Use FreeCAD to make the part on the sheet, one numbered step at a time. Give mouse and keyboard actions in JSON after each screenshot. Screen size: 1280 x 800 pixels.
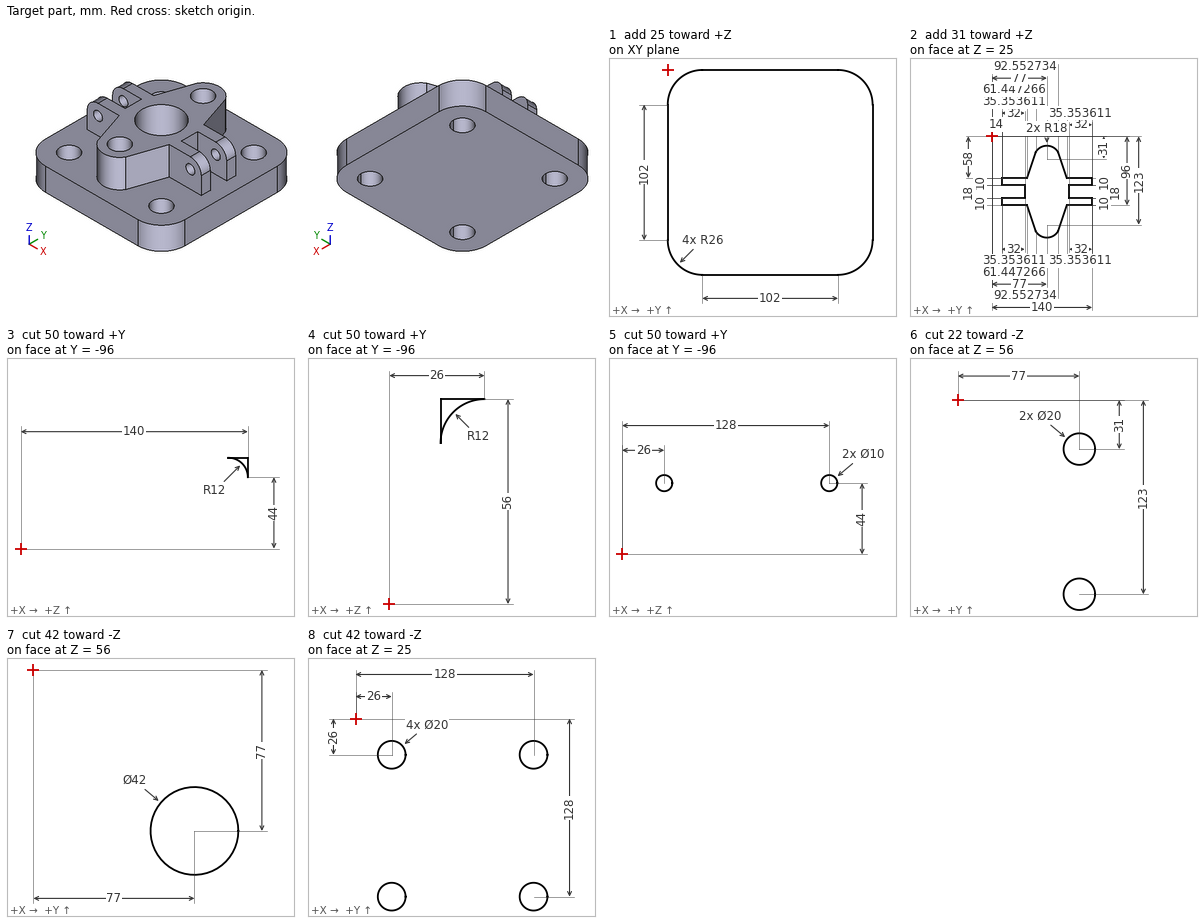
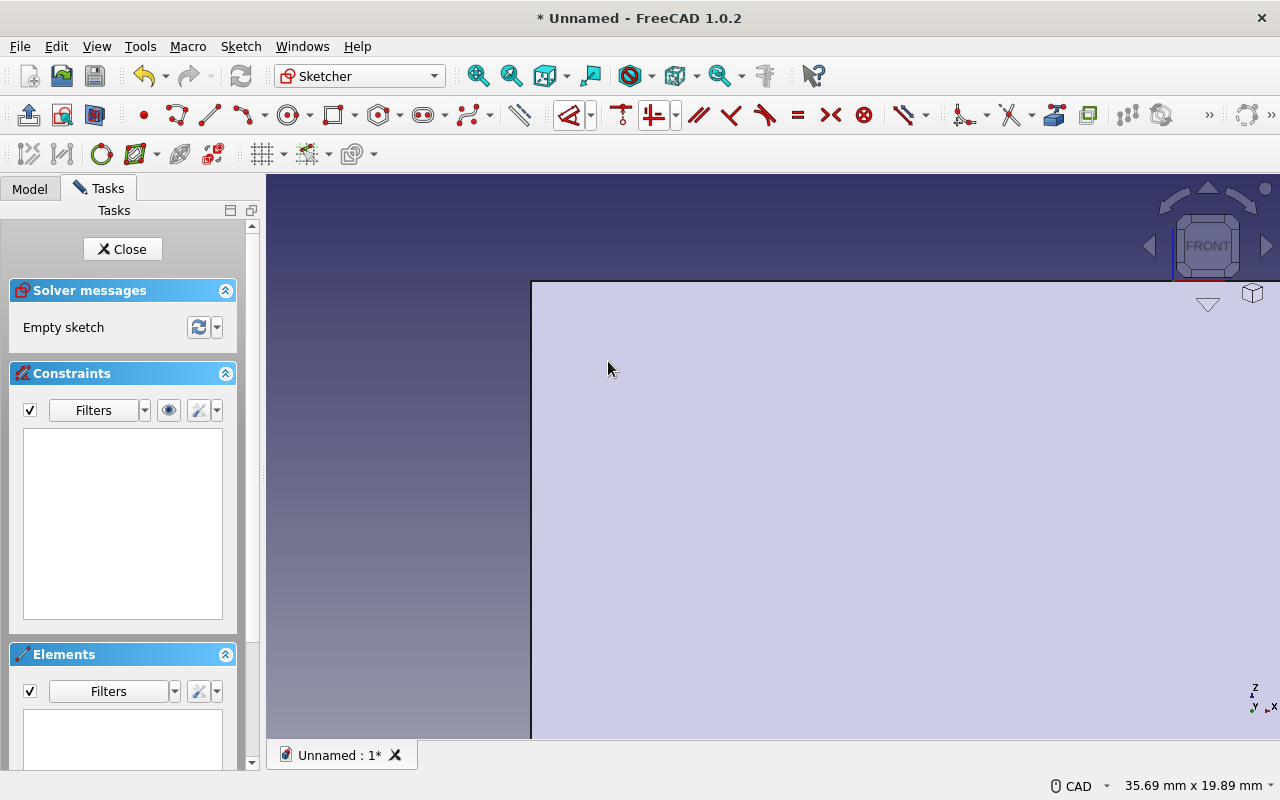
{"action": "left_click", "coordinate": [177, 116]}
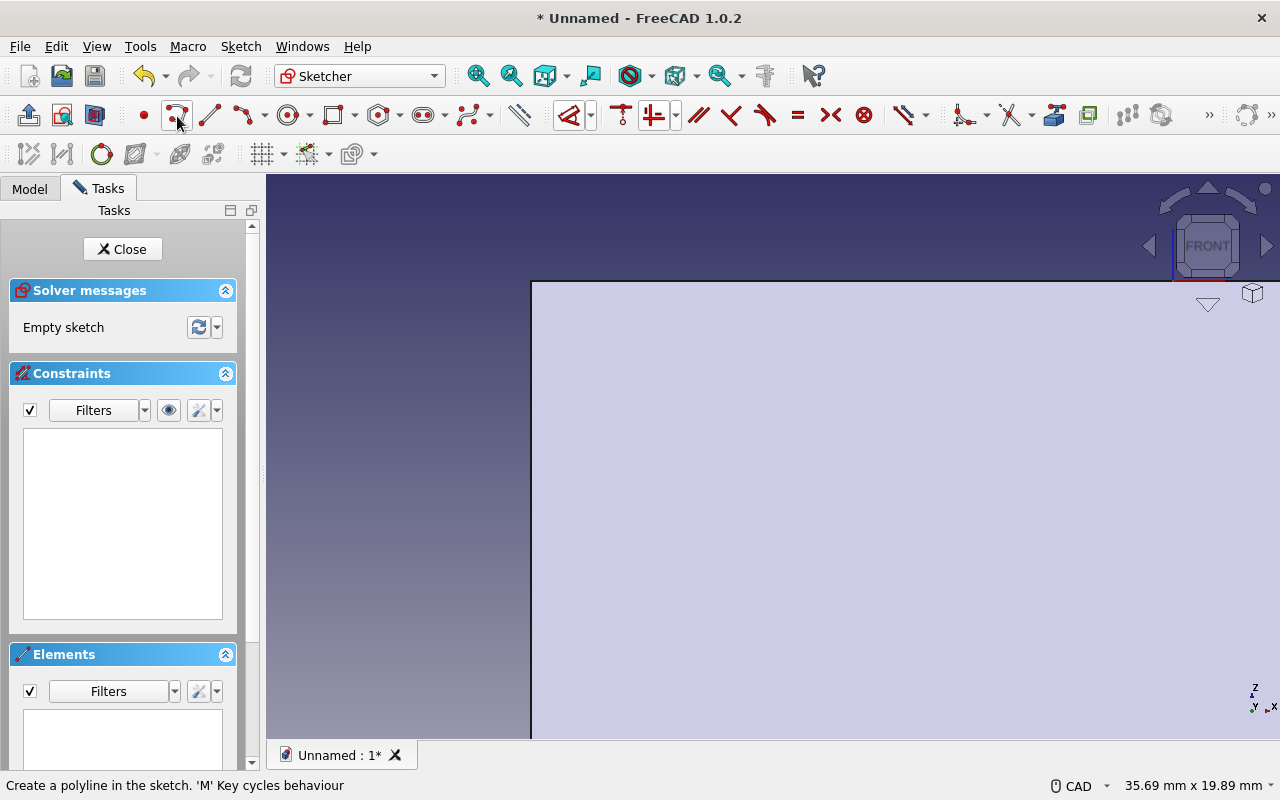
{"action": "left_click", "coordinate": [872, 281]}
{"action": "left_click", "coordinate": [531, 281]}
{"action": "left_click", "coordinate": [531, 622]}
{"action": "right_click", "coordinate": [531, 622]}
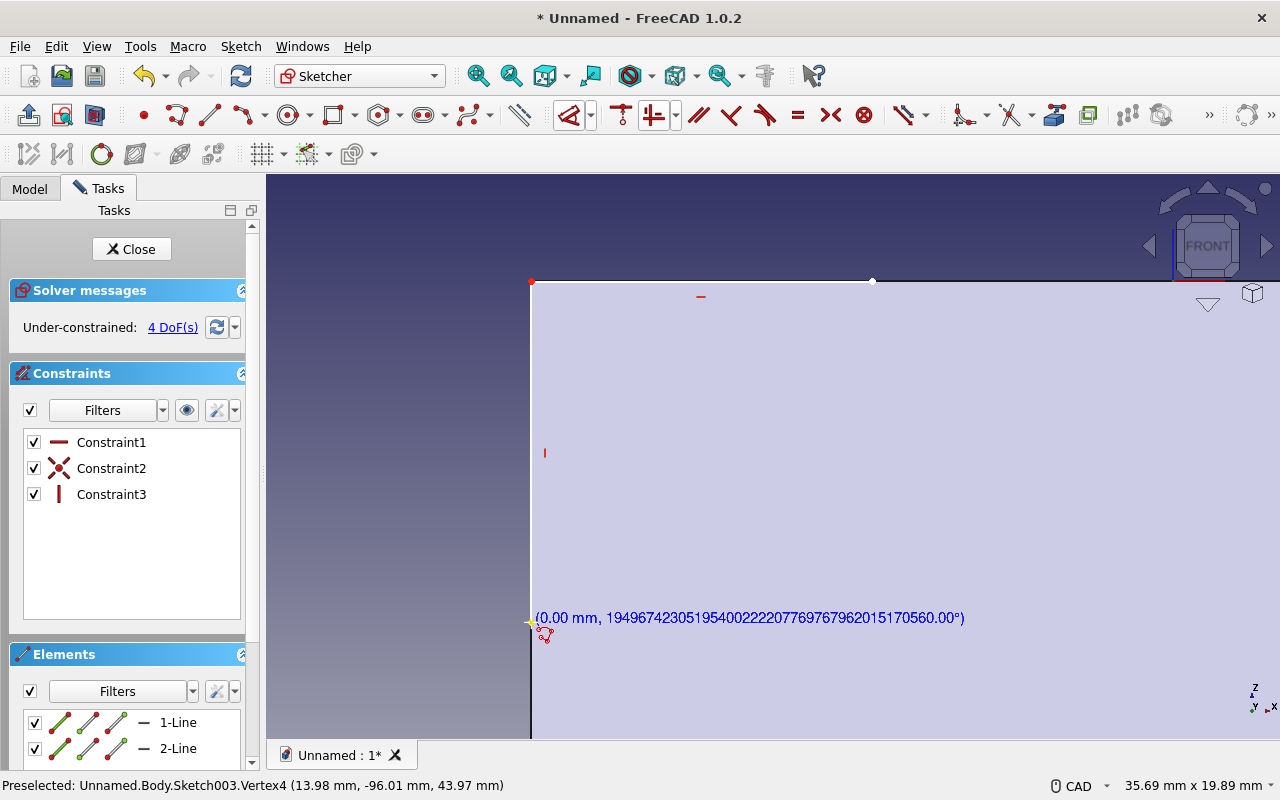
{"action": "left_click", "coordinate": [242, 116]}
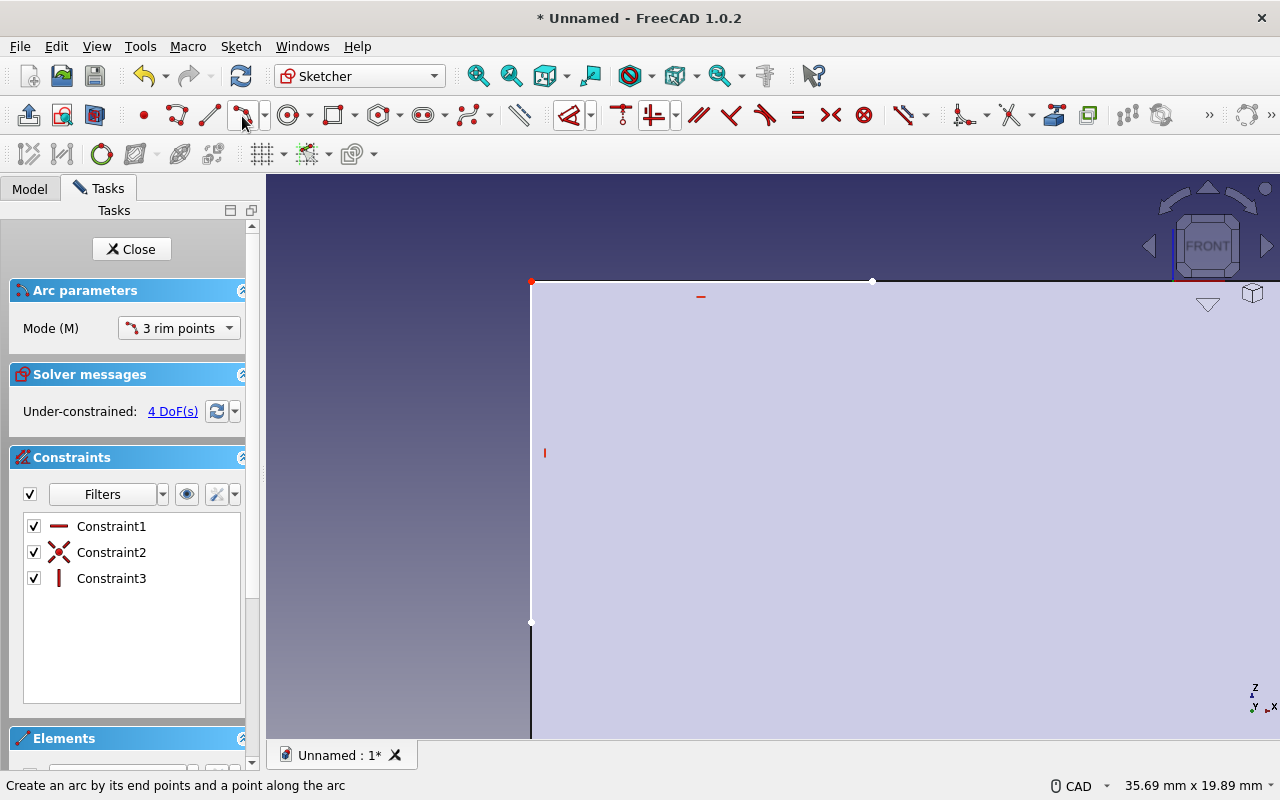
{"action": "left_click", "coordinate": [531, 623]}
{"action": "left_click", "coordinate": [872, 282]}
{"action": "left_click", "coordinate": [631, 381]}
{"action": "key", "text": "Escape"}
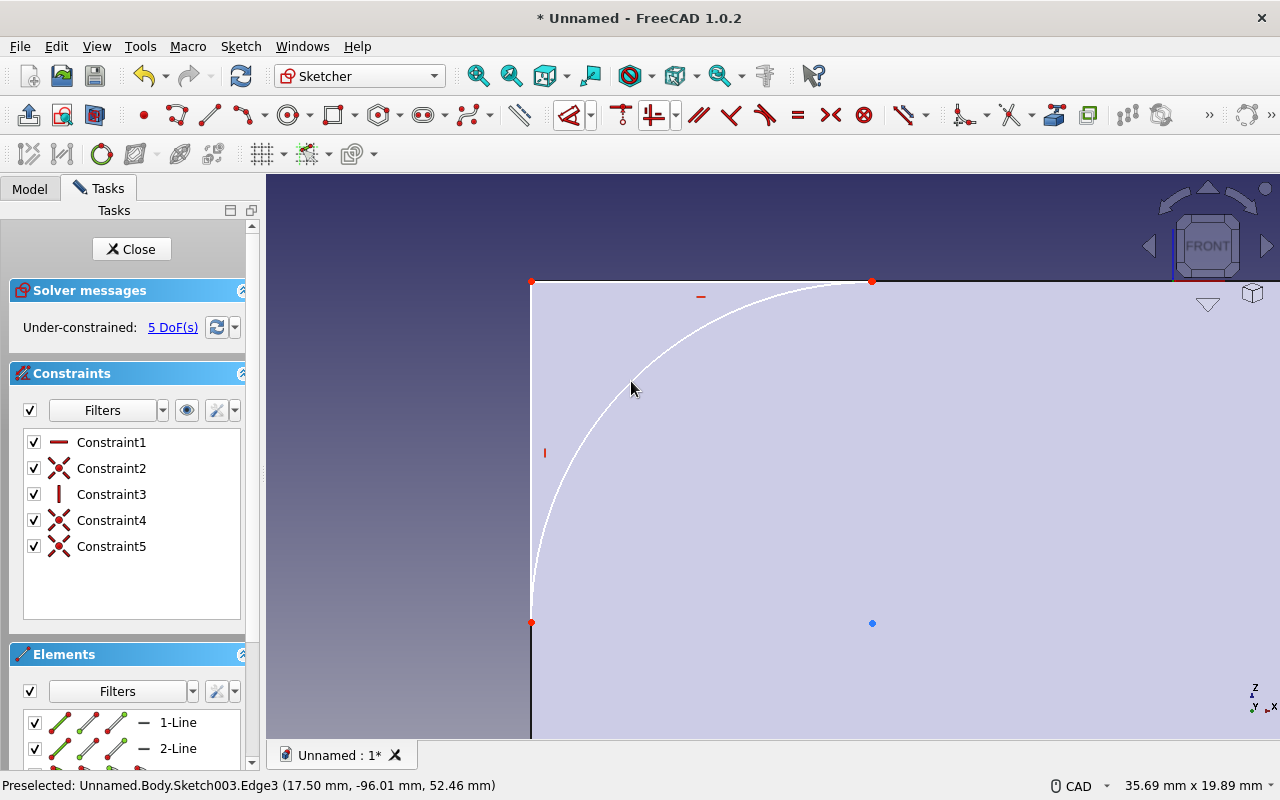
{"action": "left_click", "coordinate": [770, 282]}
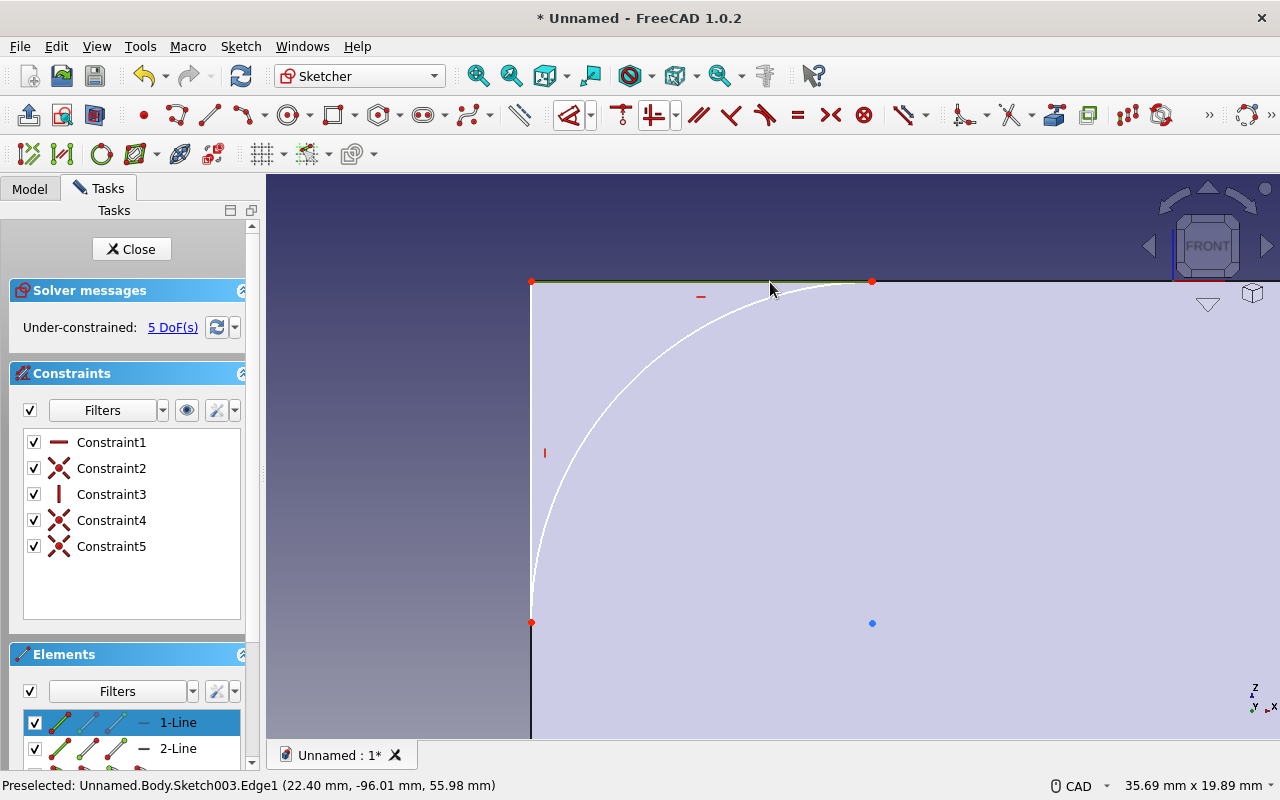
{"action": "left_click", "coordinate": [717, 319]}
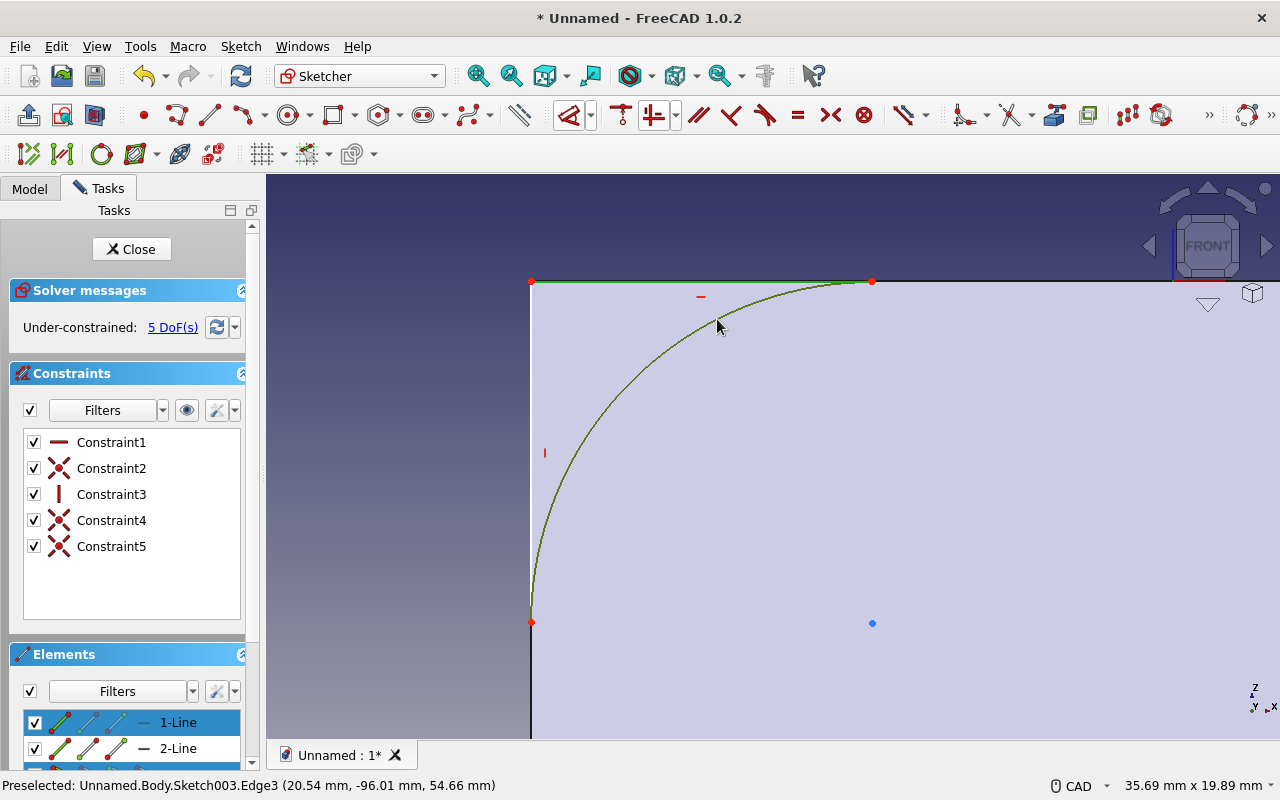
{"action": "left_click", "coordinate": [765, 116]}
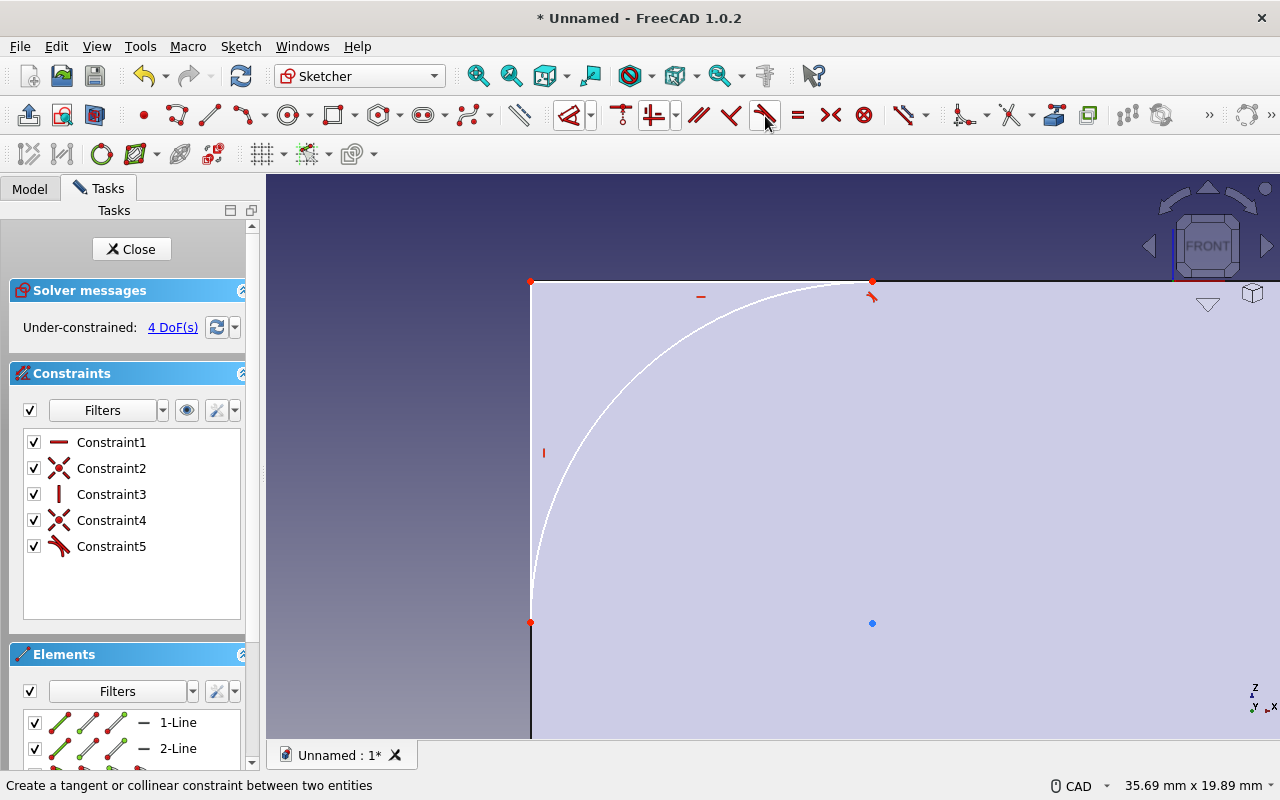
{"action": "left_click", "coordinate": [531, 384]}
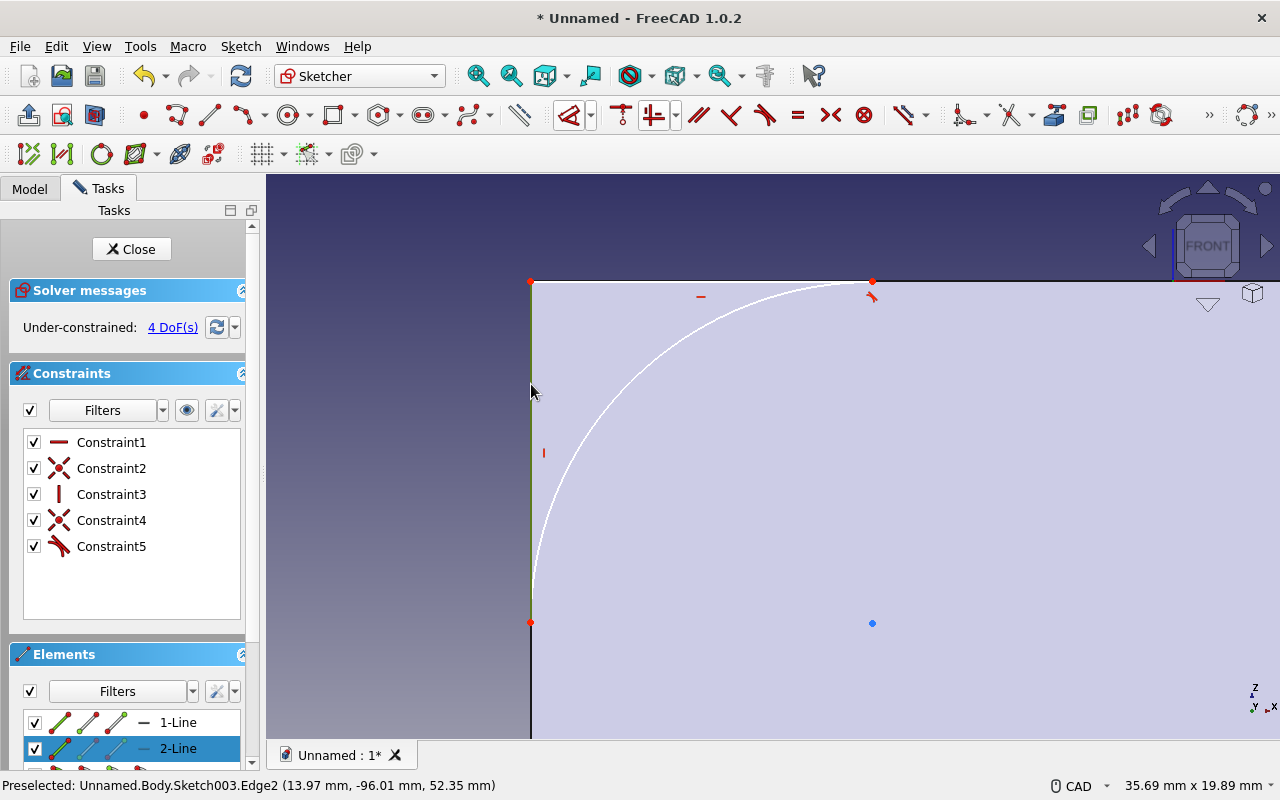
{"action": "left_click", "coordinate": [717, 319]}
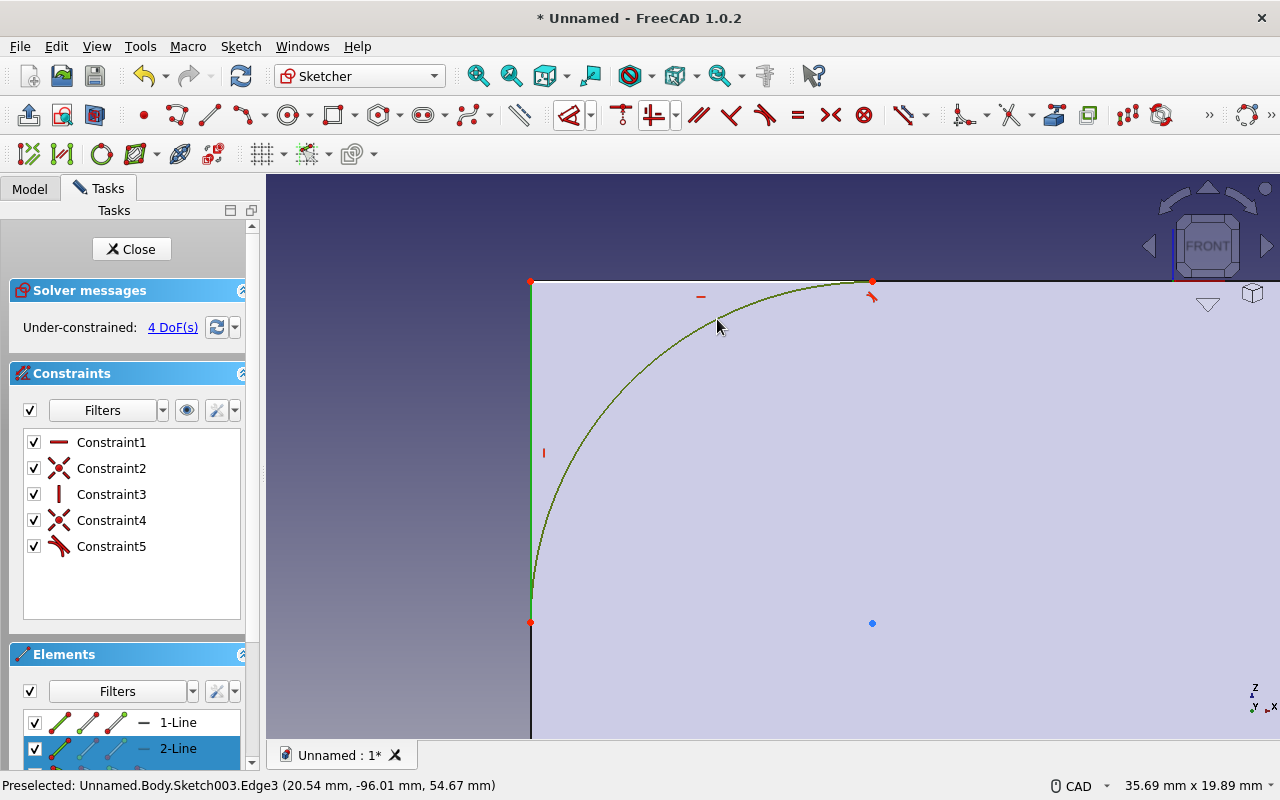
{"action": "left_click", "coordinate": [765, 116]}